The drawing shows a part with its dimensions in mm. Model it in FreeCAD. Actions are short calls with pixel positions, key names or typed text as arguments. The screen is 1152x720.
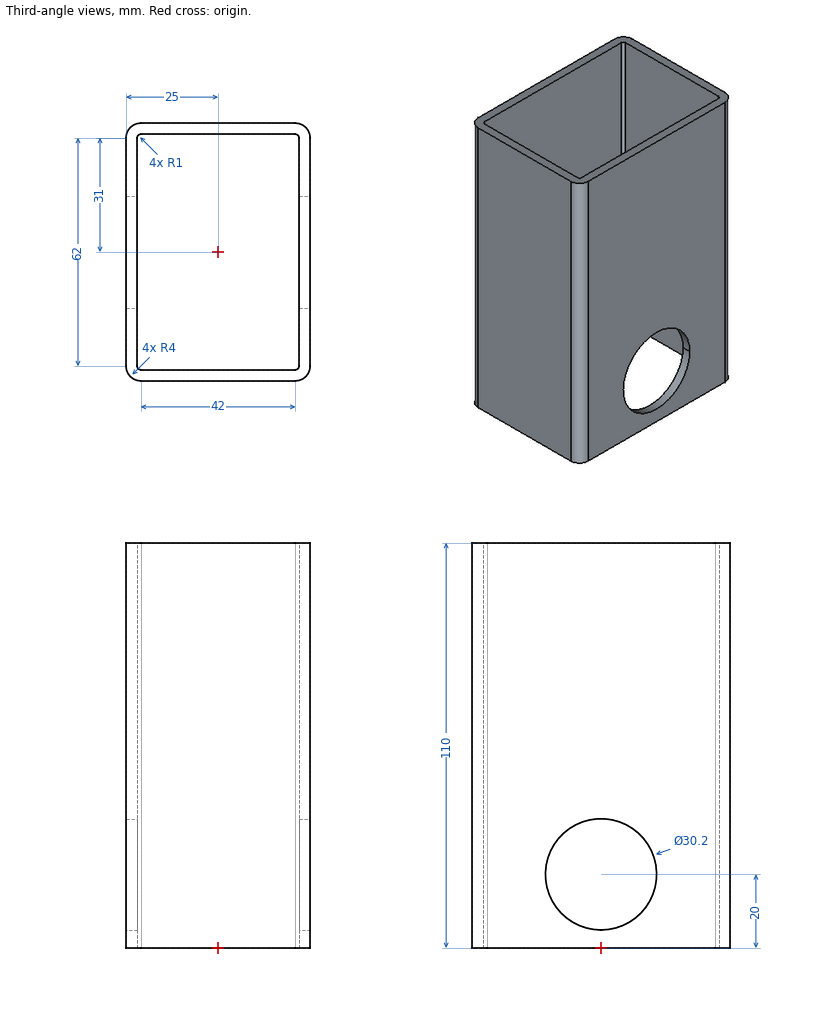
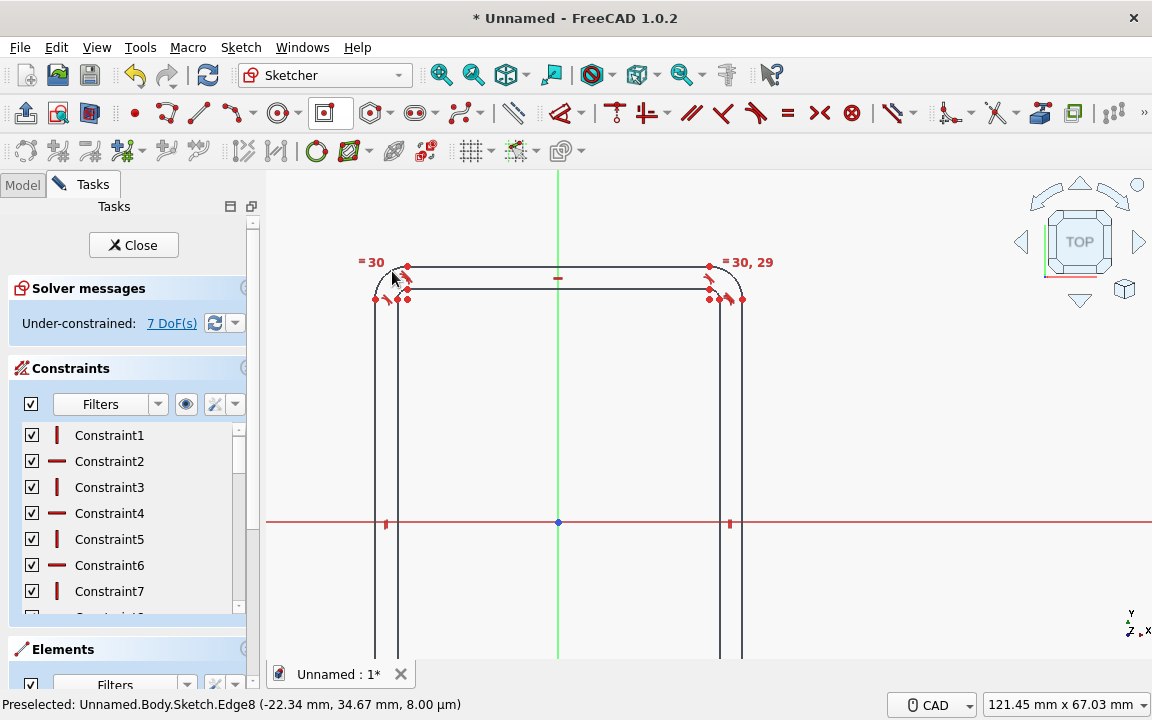
scroll(401, 292, up, 4)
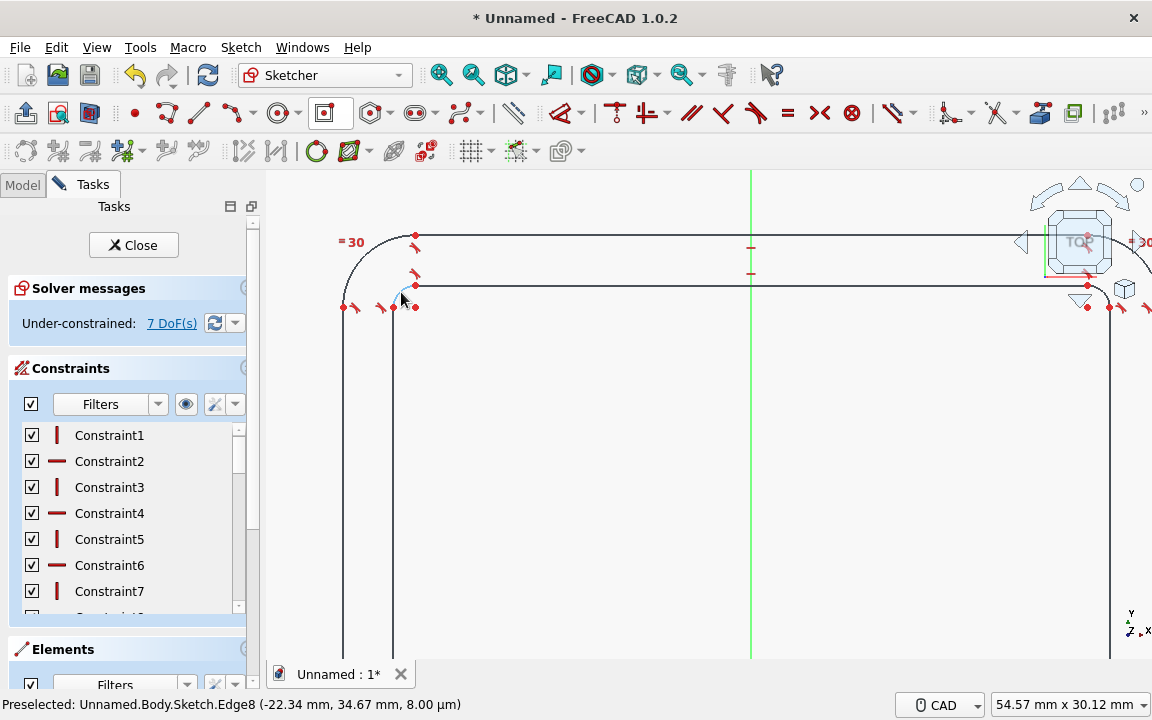
click(400, 292)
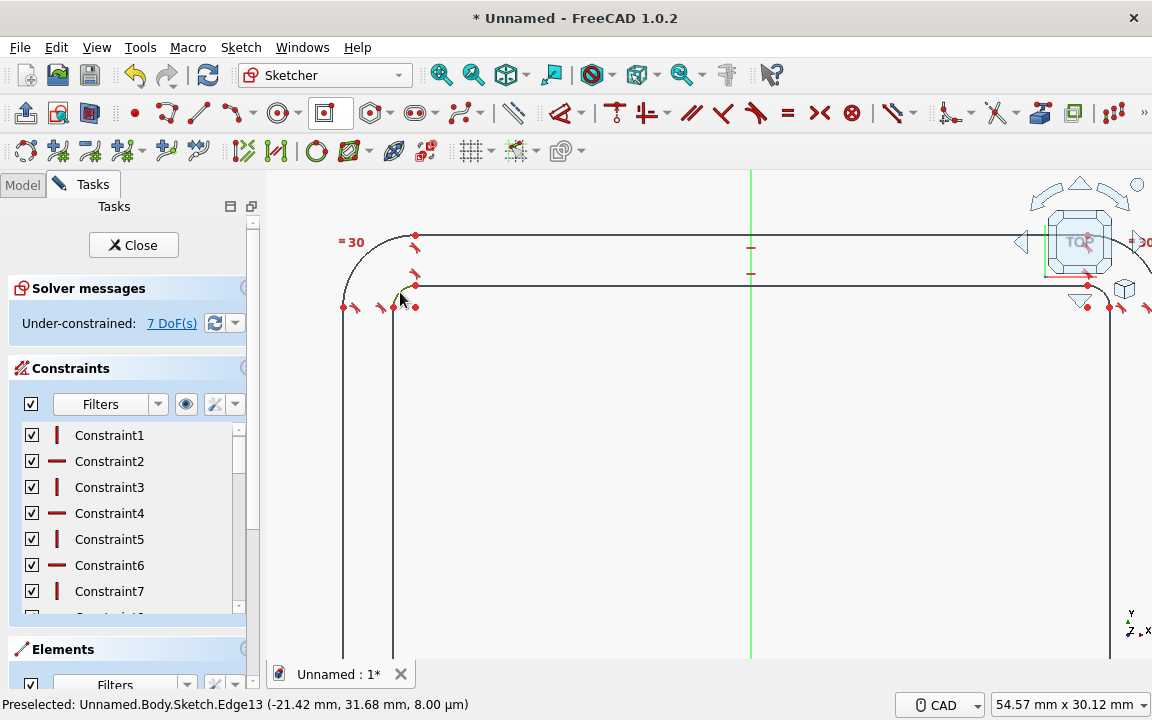
scroll(604, 287, down, 7)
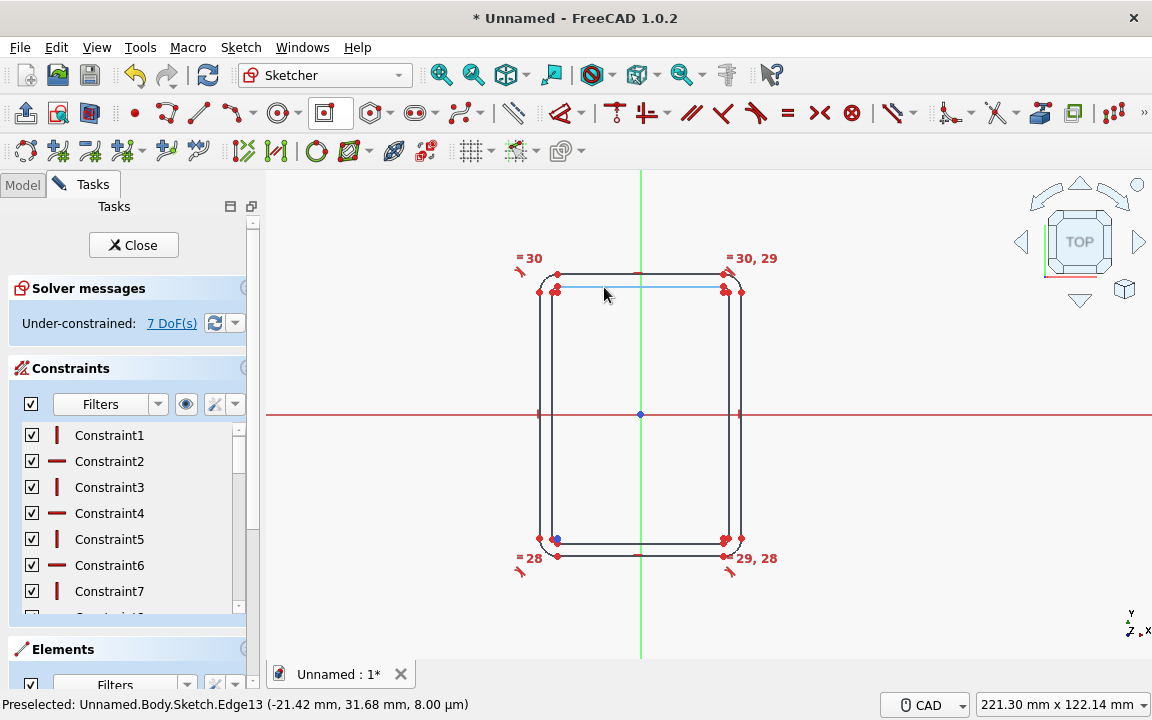
scroll(553, 541, up, 10)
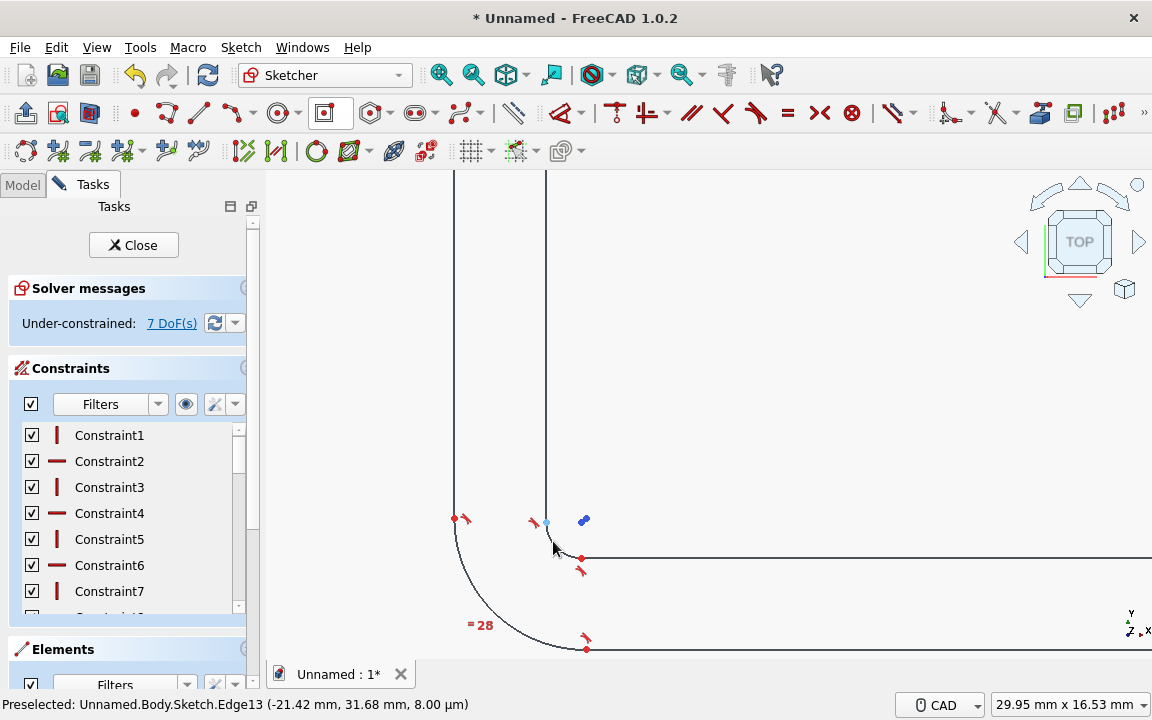
click(550, 539)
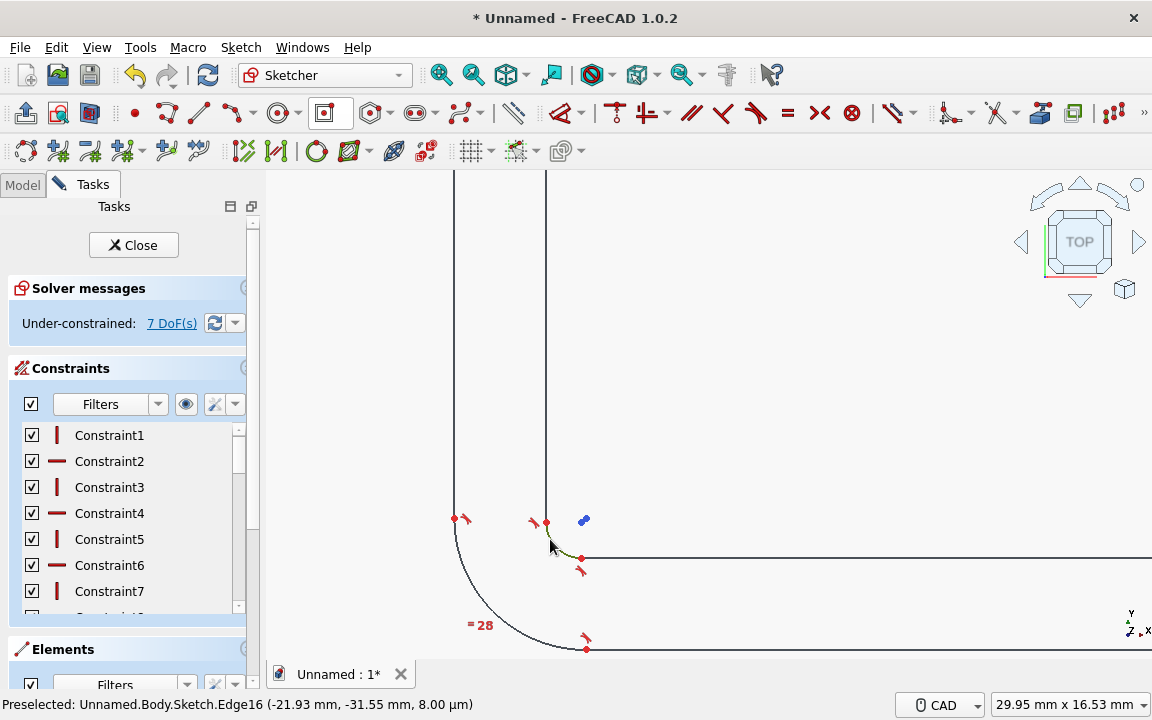
key(e)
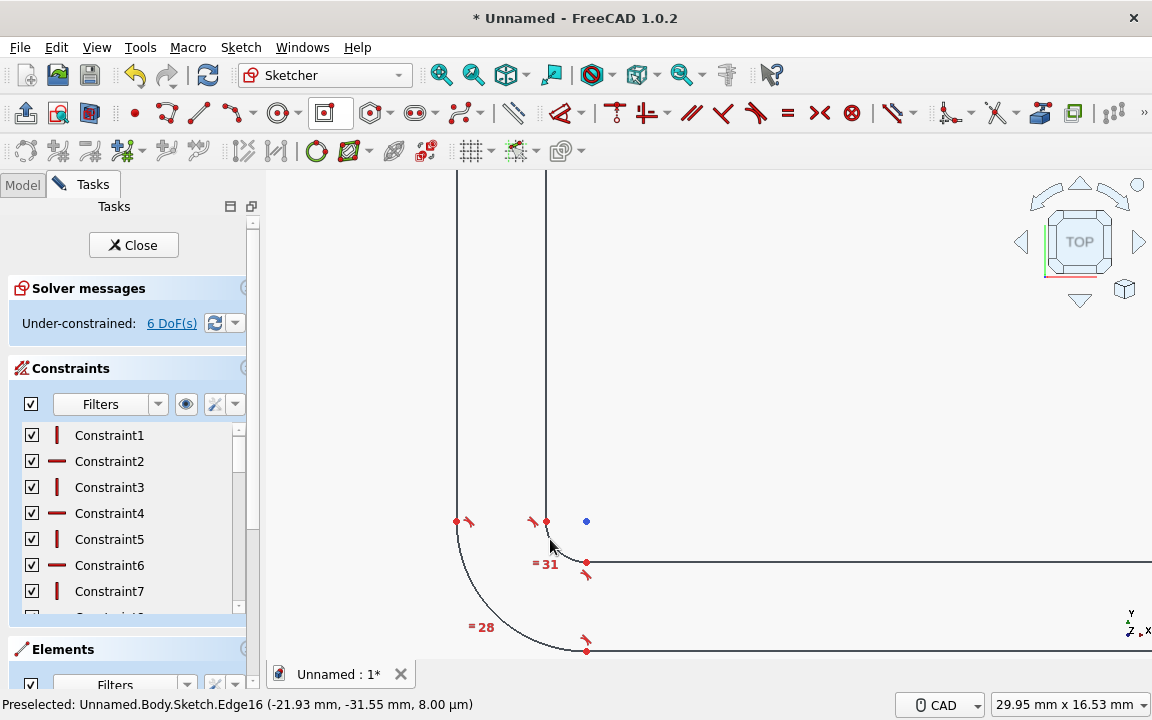
key(d)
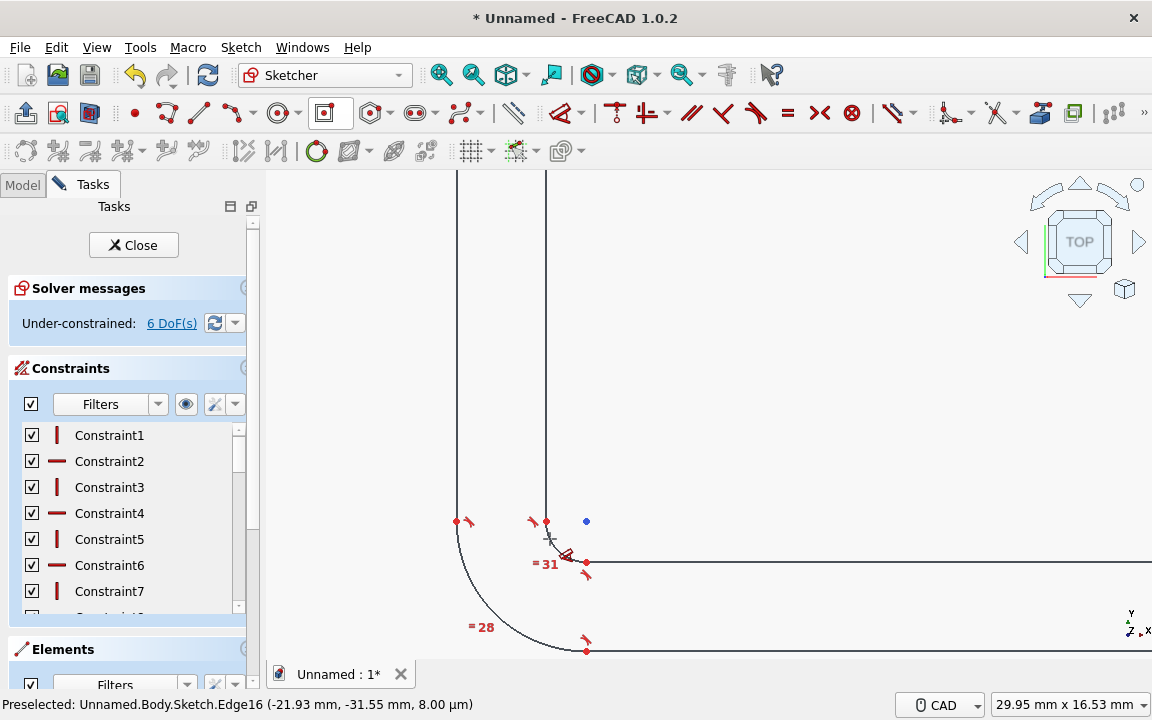
scroll(553, 542, down, 10)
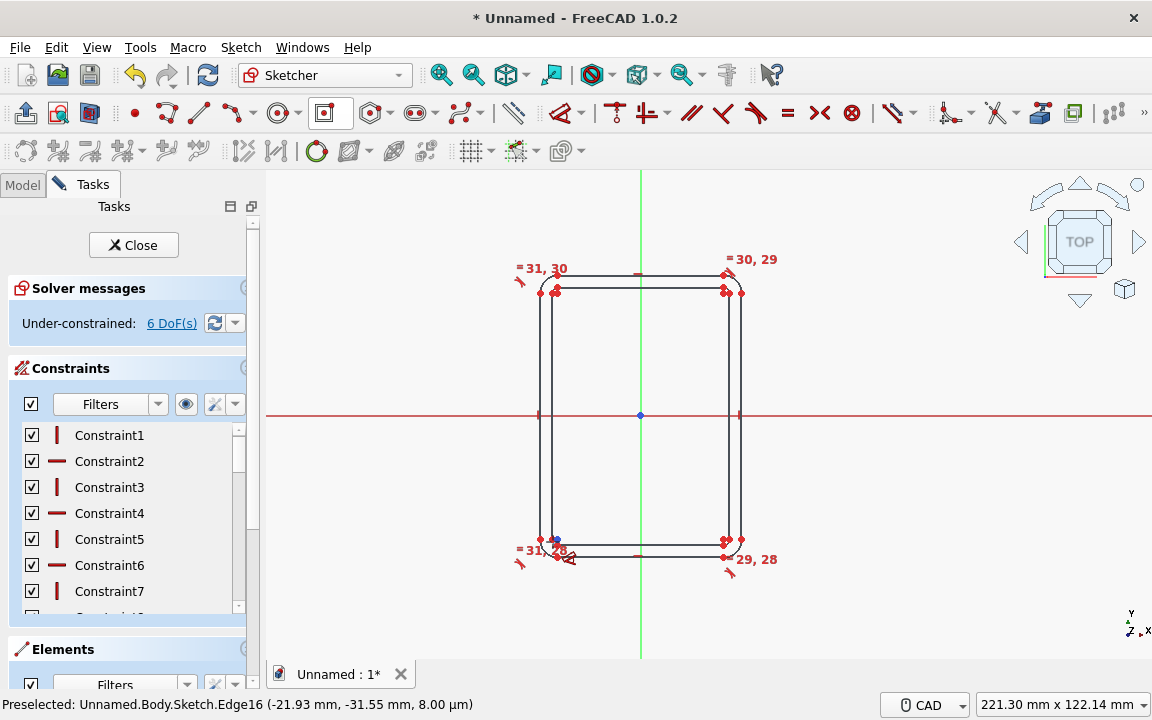
scroll(542, 548, up, 5)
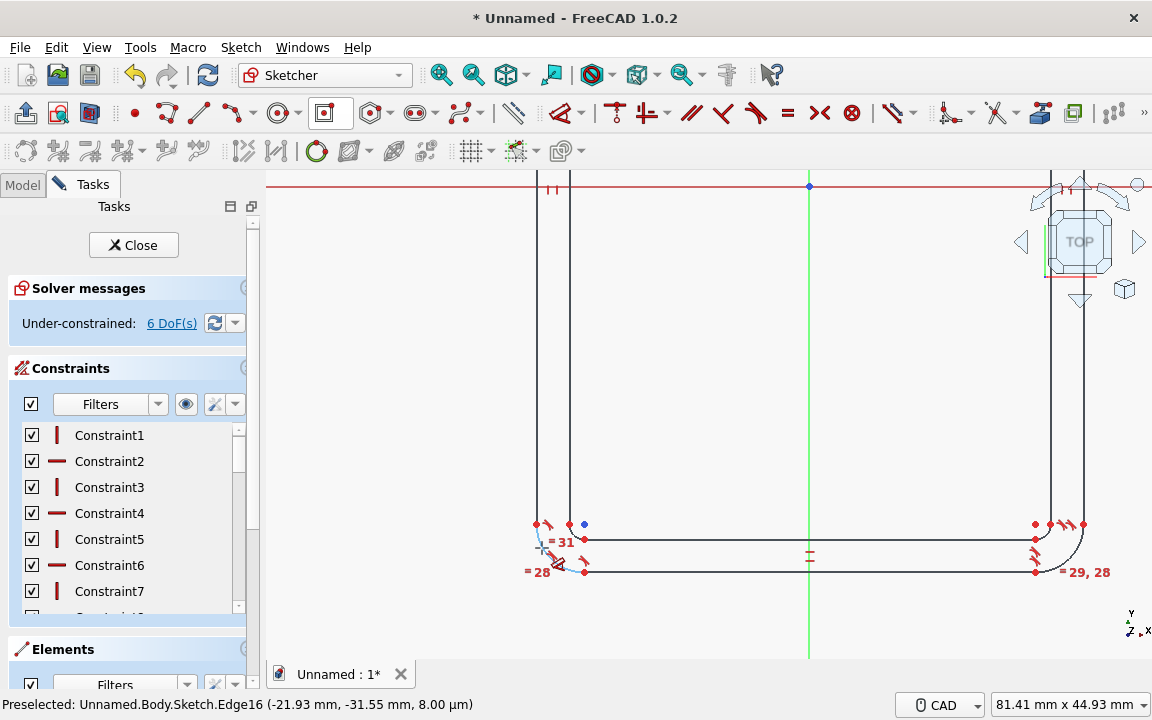
click(542, 546)
click(513, 560)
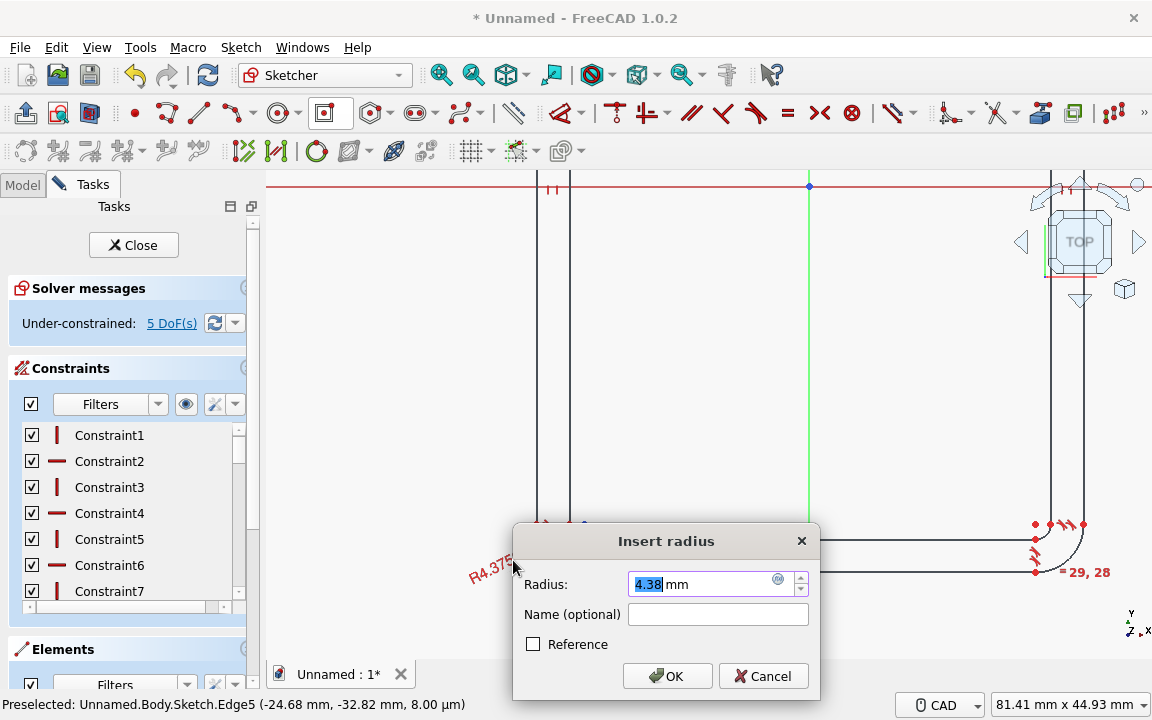
text(4)
key(Return)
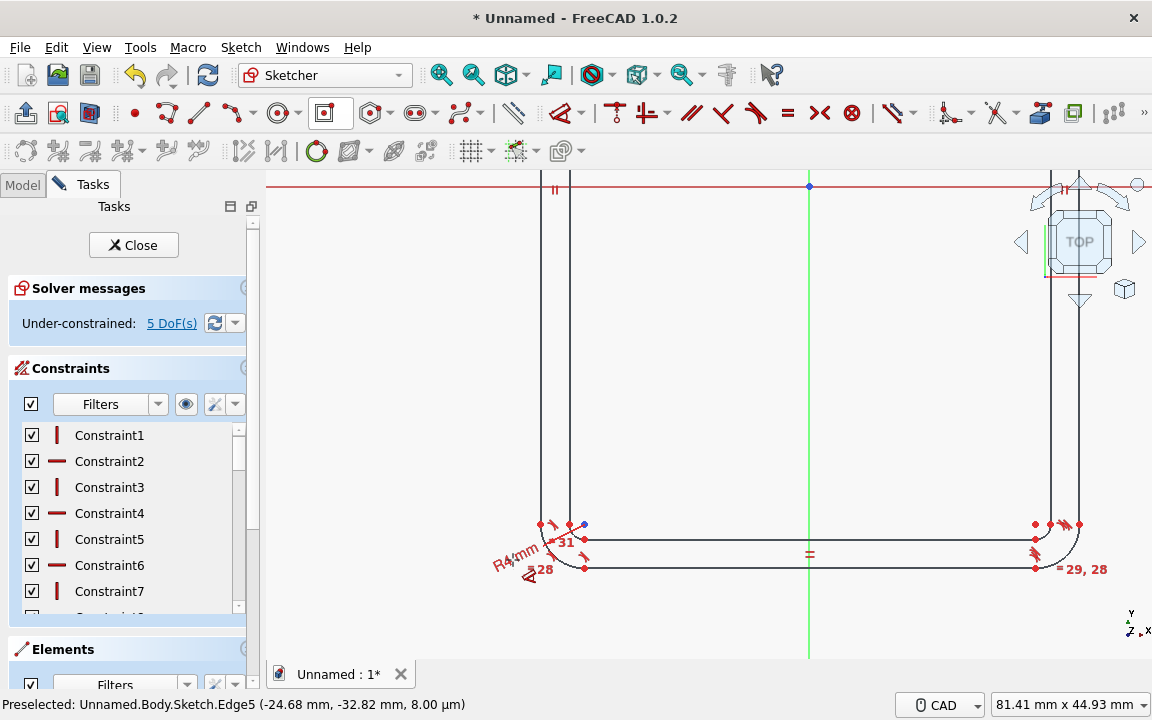
scroll(542, 547, down, 5)